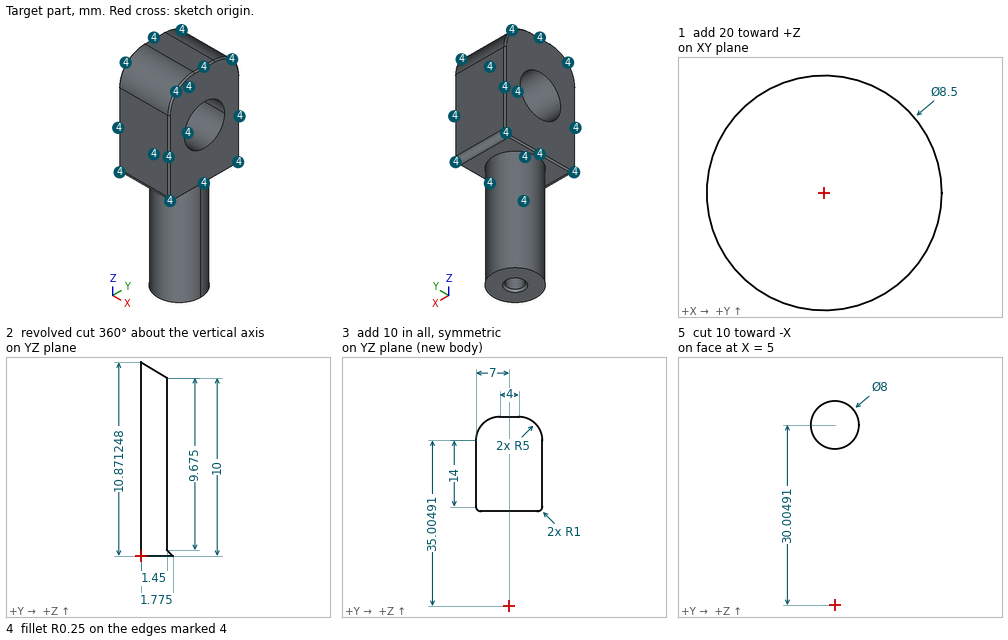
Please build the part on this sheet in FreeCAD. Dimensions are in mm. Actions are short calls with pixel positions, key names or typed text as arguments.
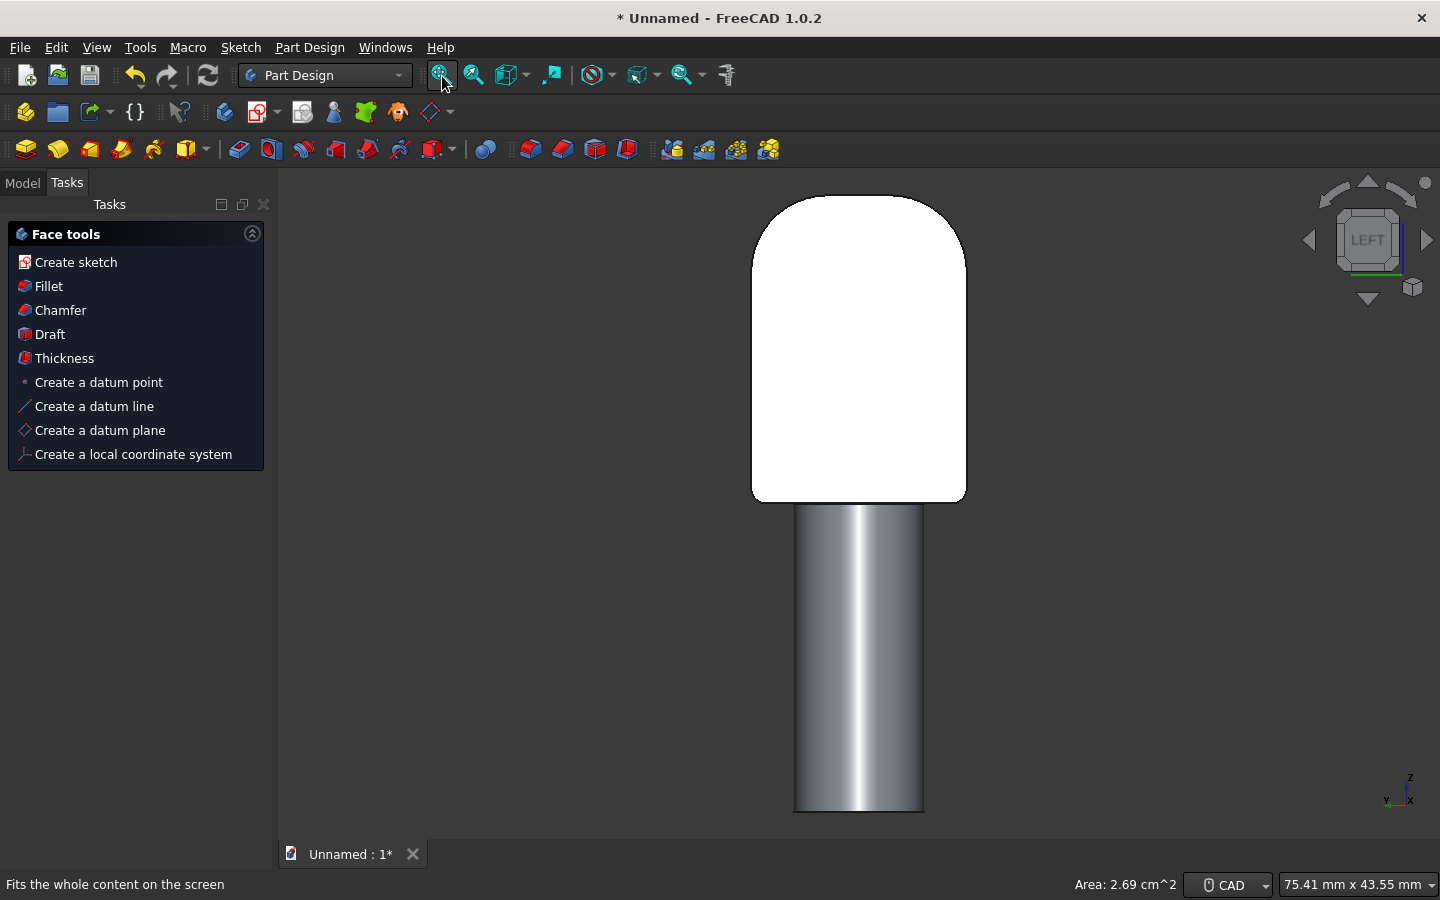
click(859, 392, ctrl)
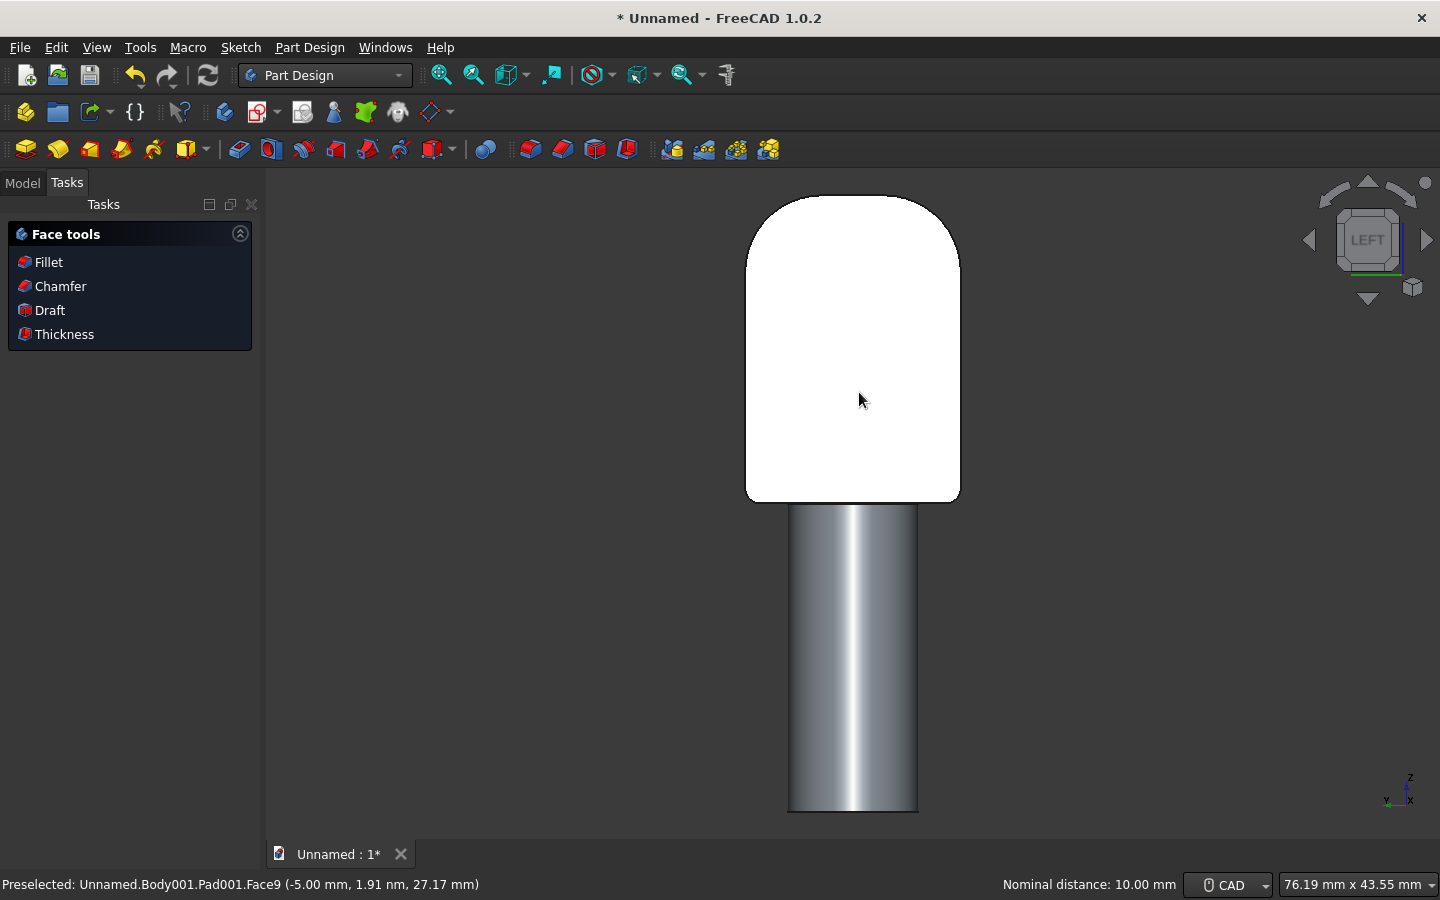
click(532, 150)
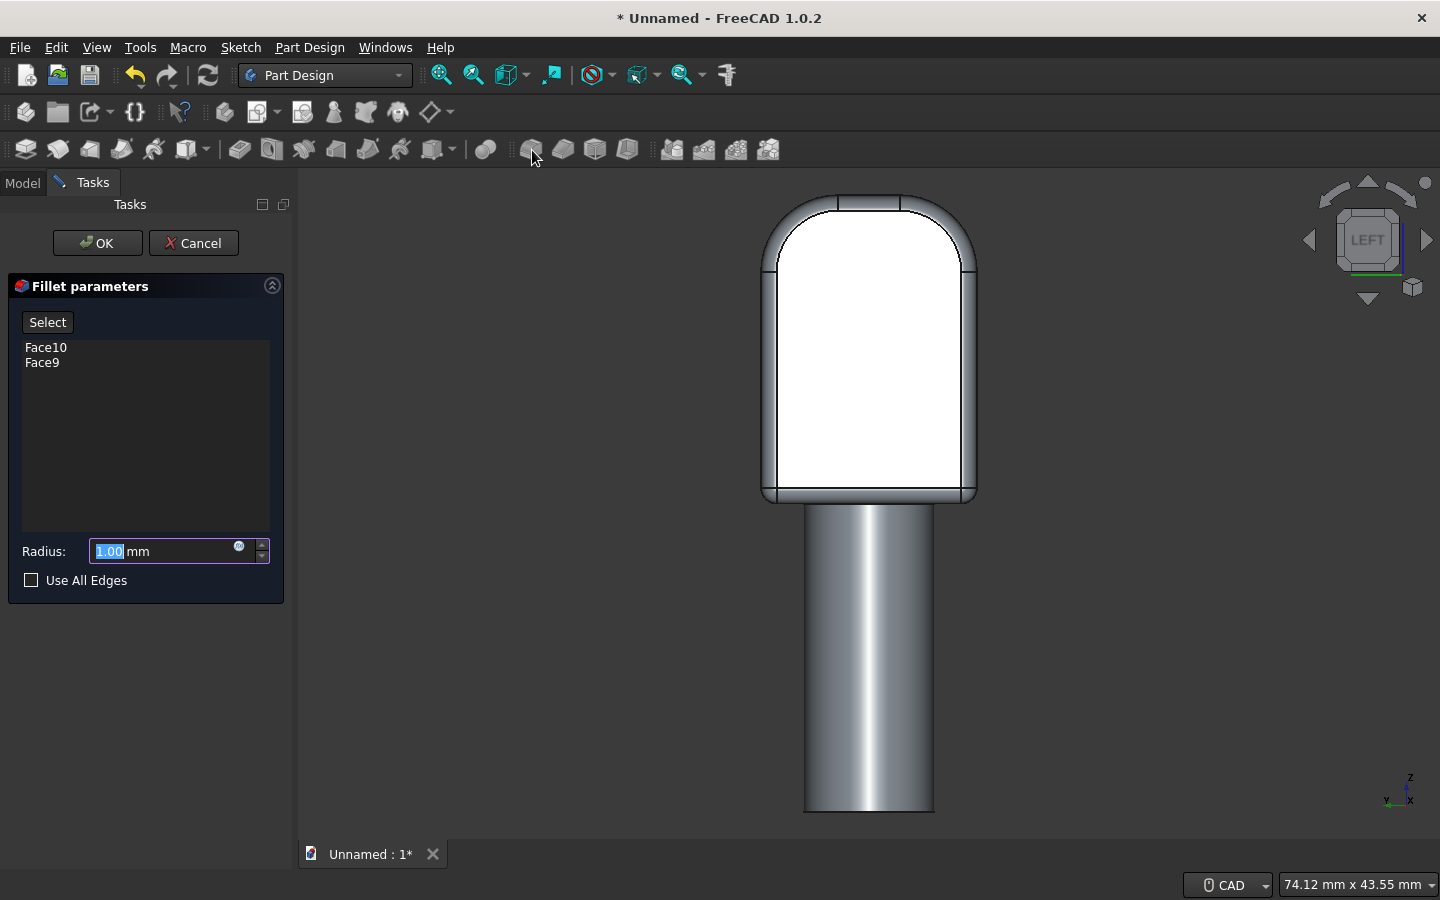
text(0.25)
key(Tab)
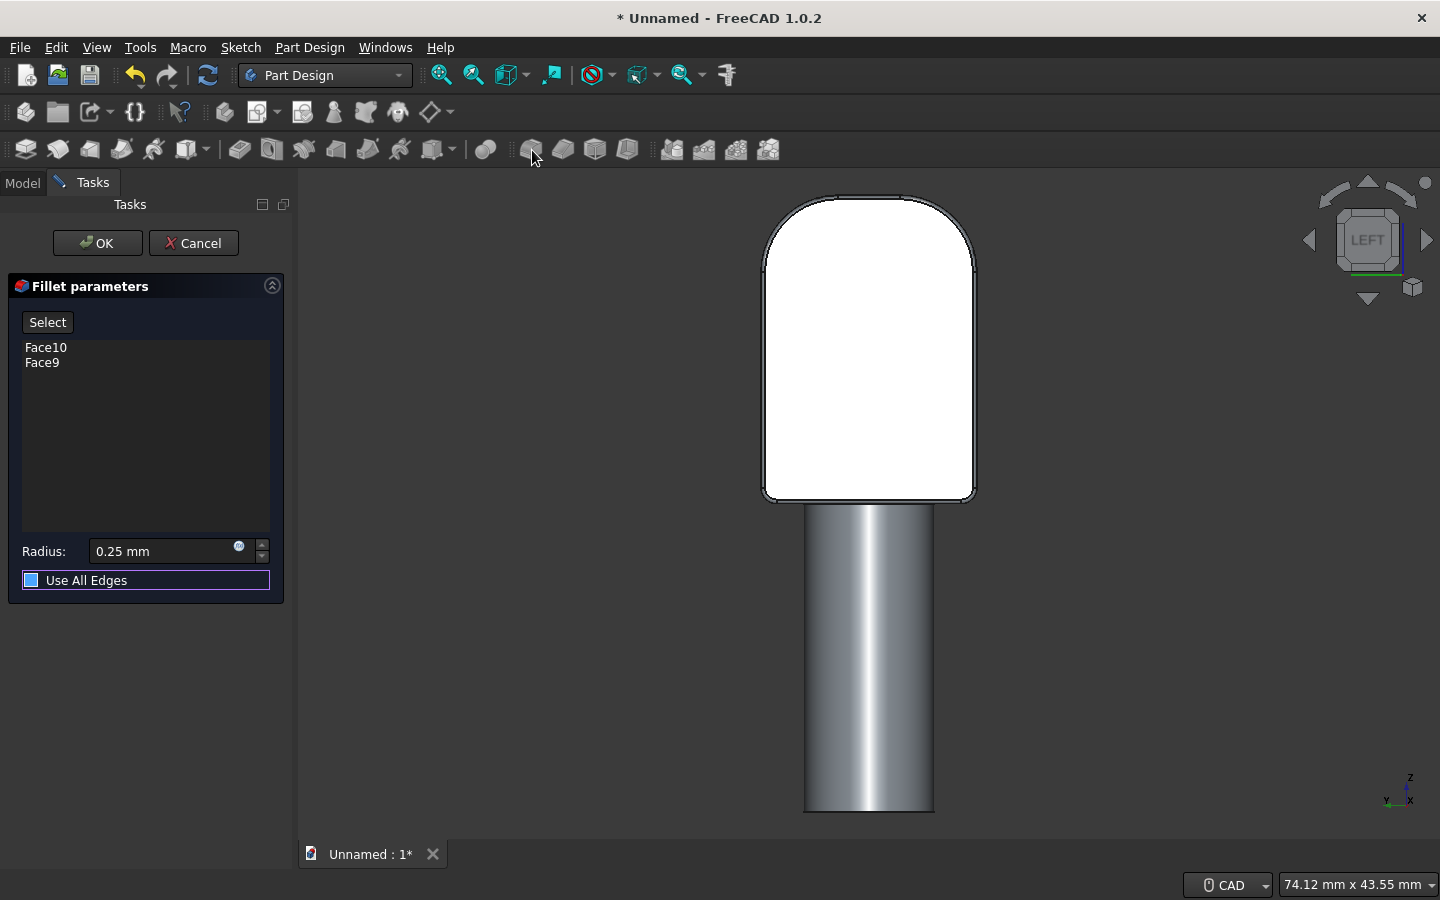
click(98, 243)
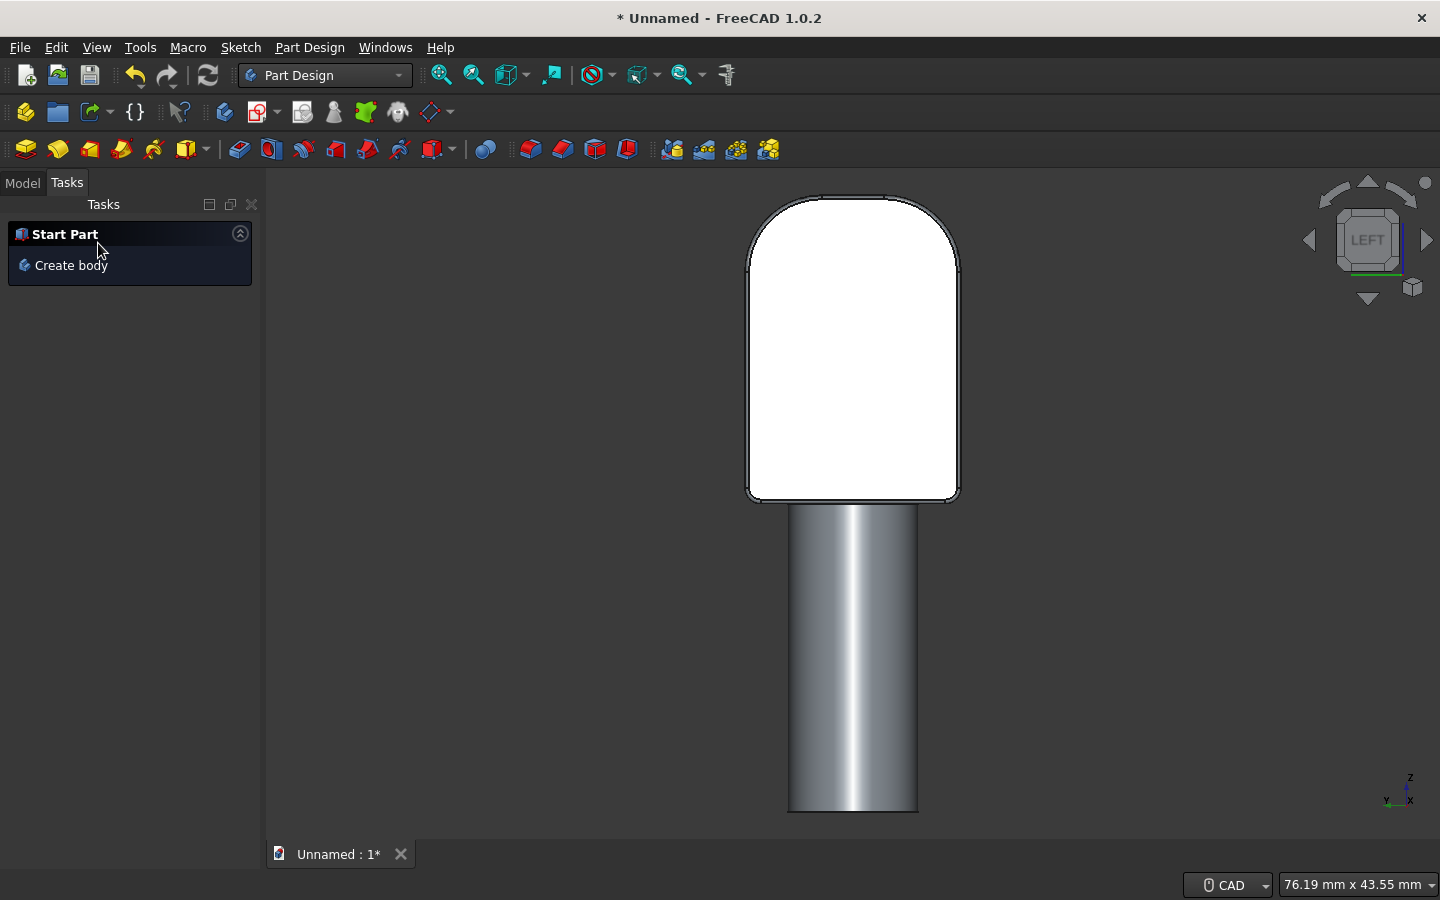
key(0)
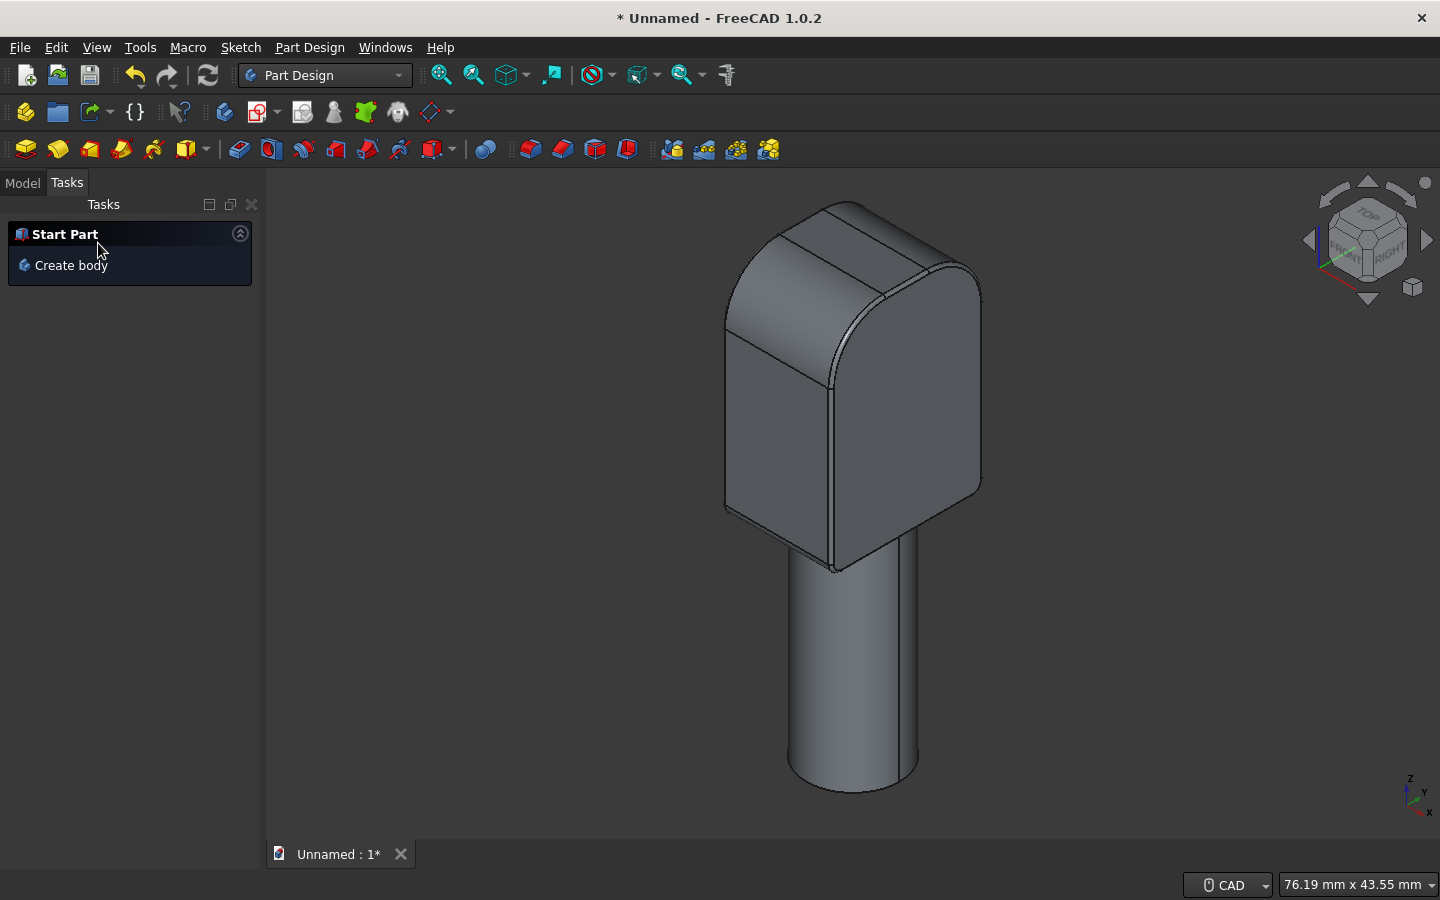
click(907, 443)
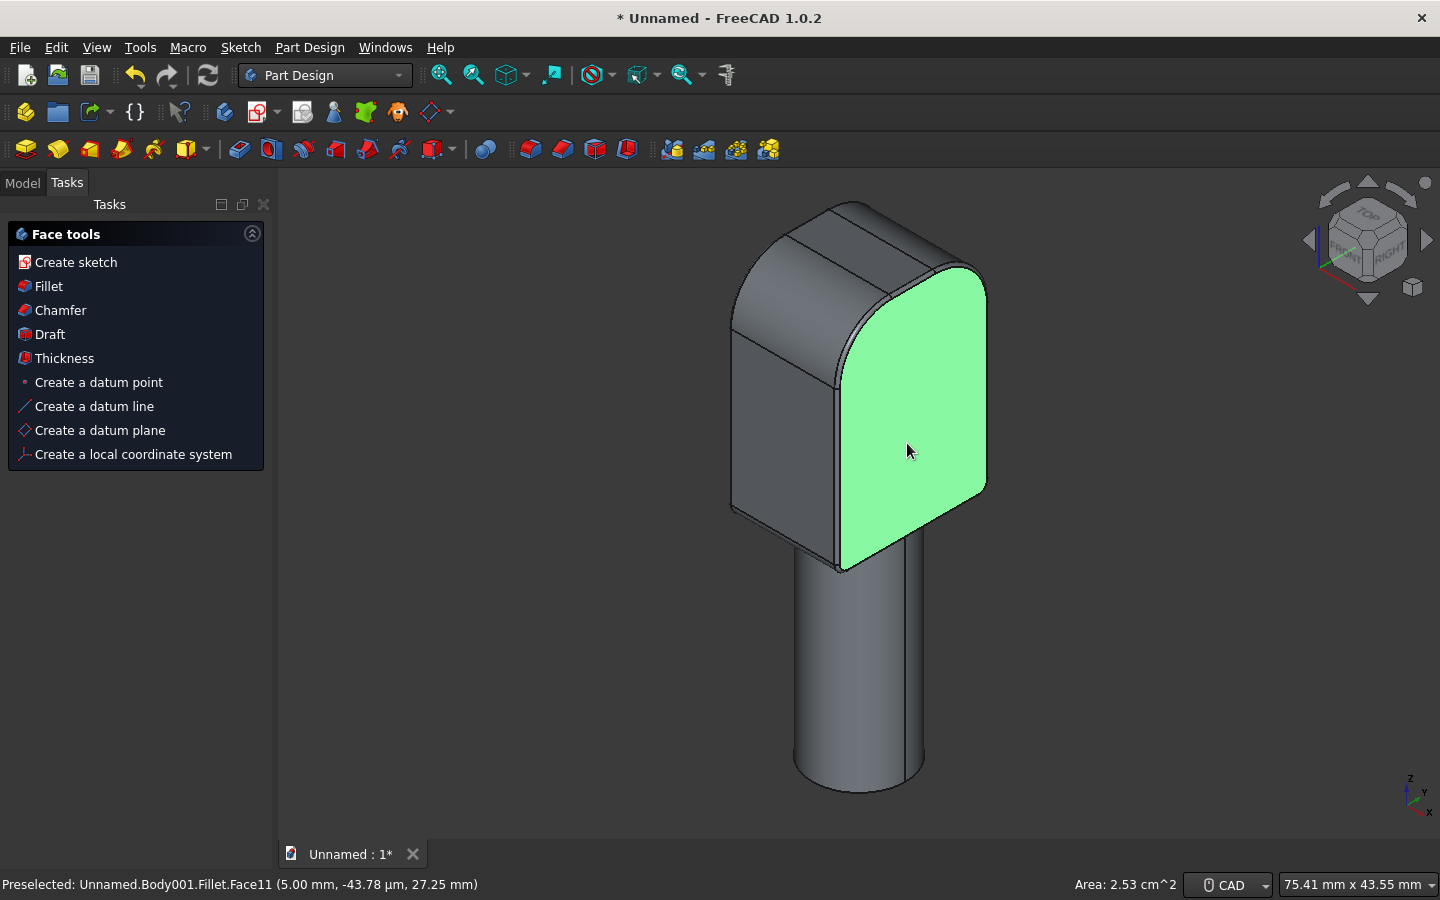
click(258, 112)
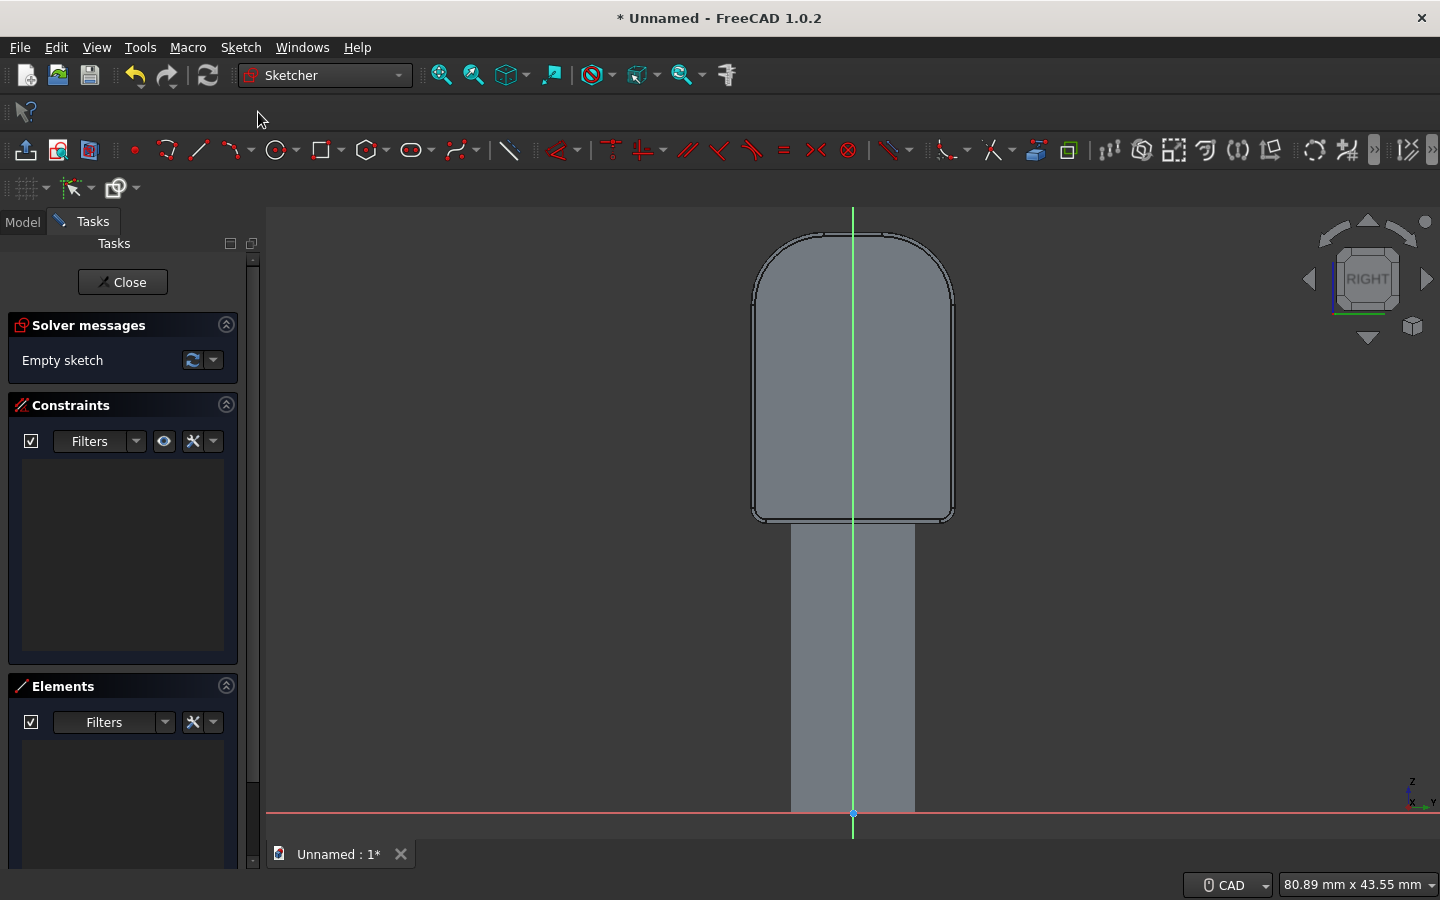
scroll(883, 315, up, 6)